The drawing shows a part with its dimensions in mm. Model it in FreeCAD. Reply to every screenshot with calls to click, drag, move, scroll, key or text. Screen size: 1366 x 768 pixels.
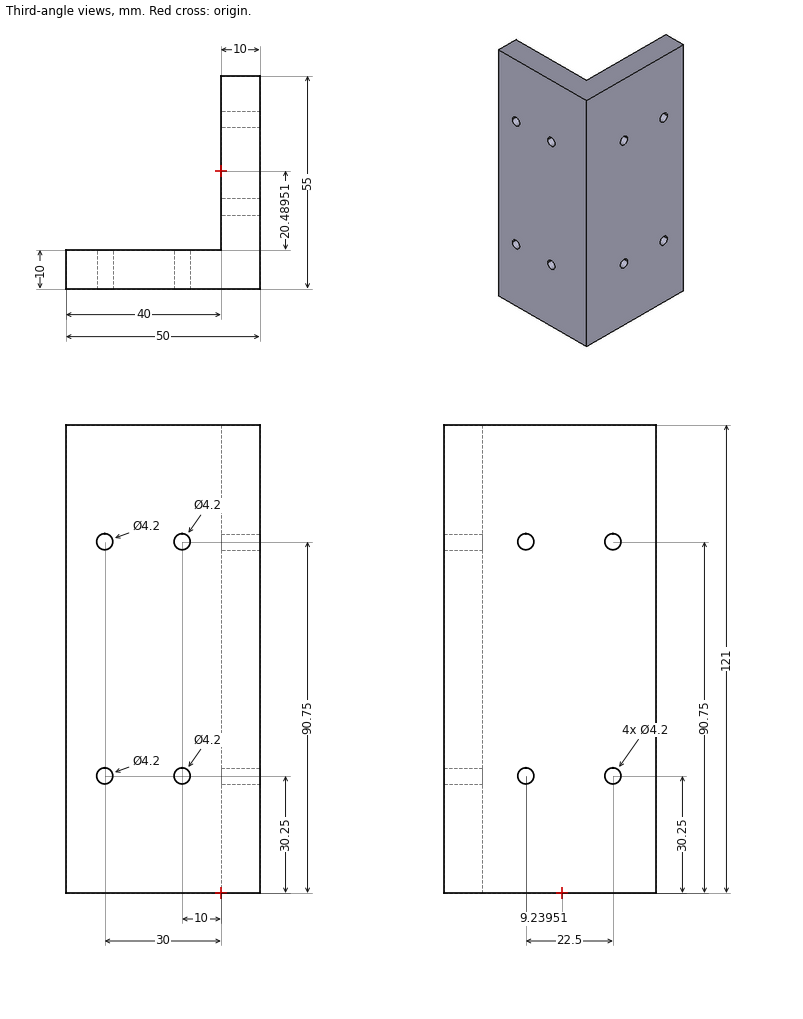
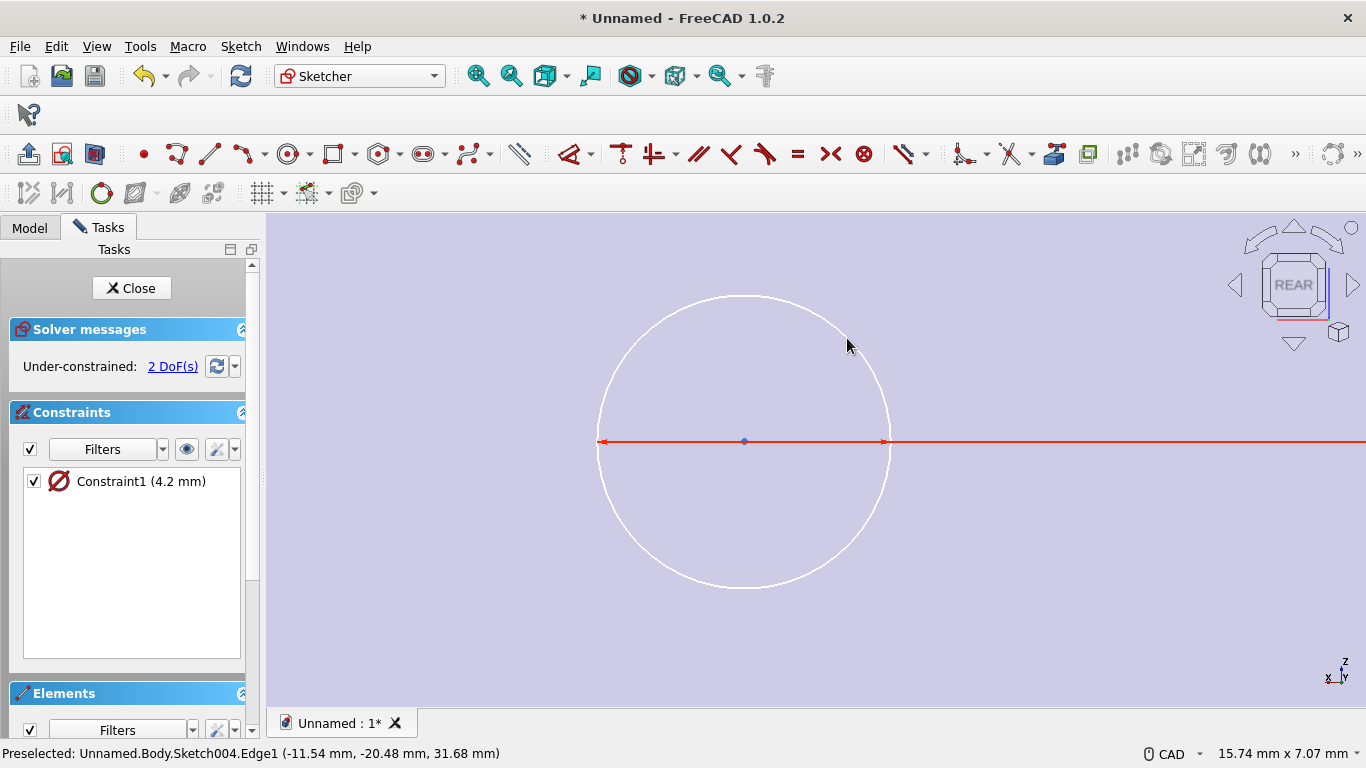
key(d)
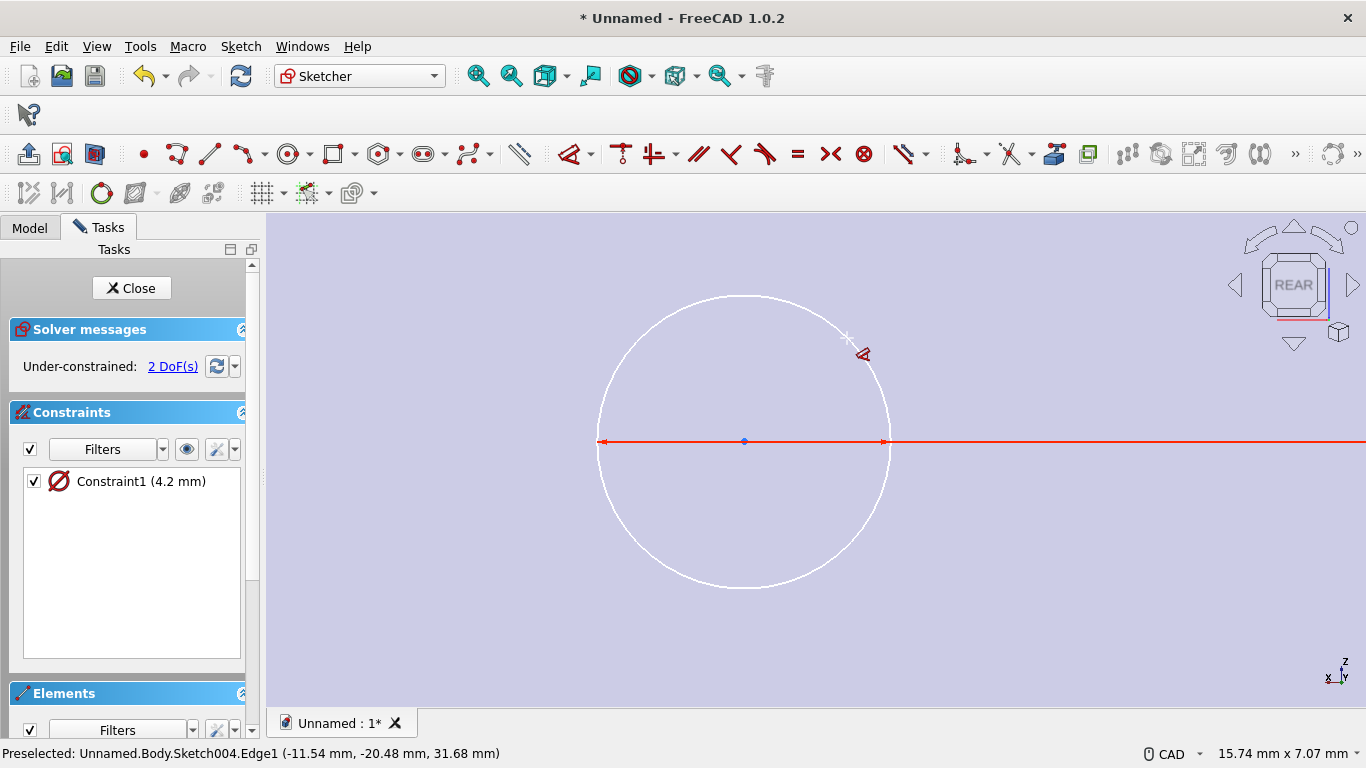
click(744, 442)
click(519, 408)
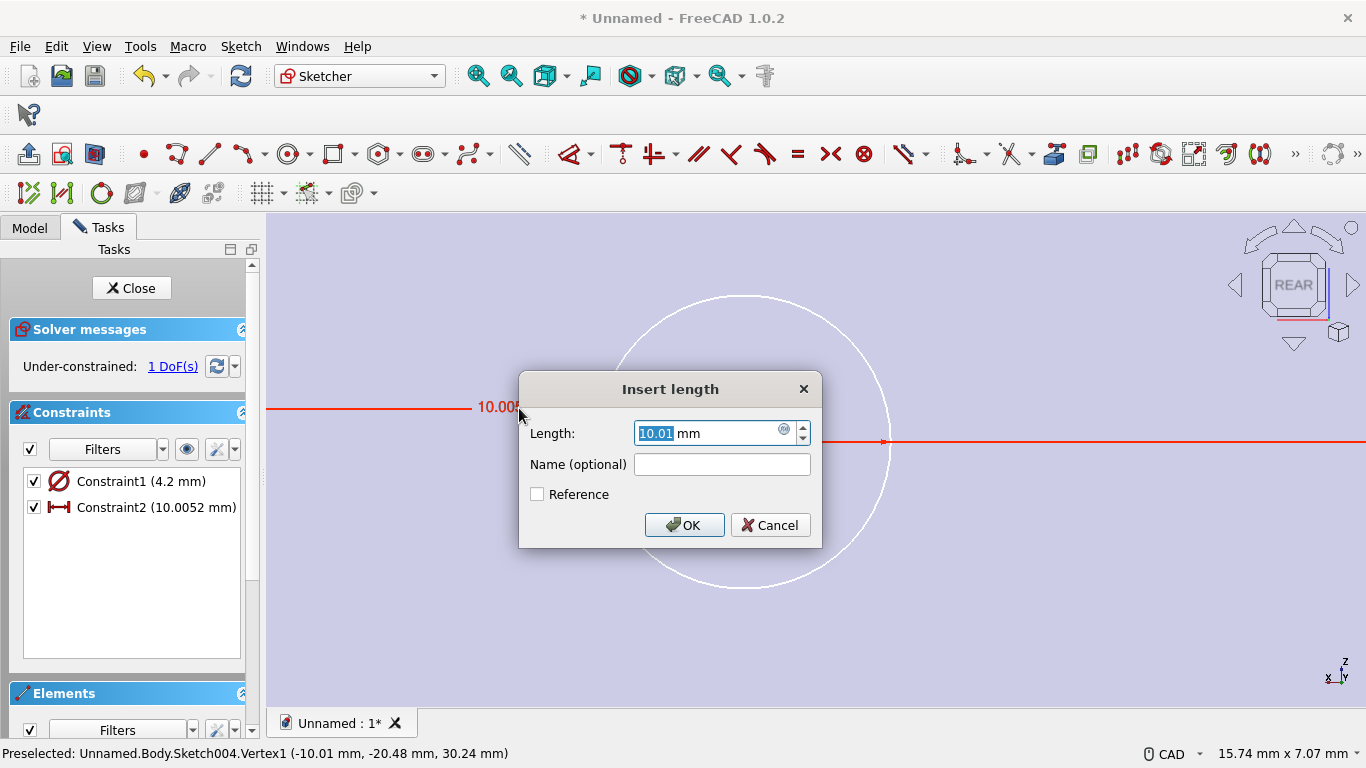
text(10)
key(Return)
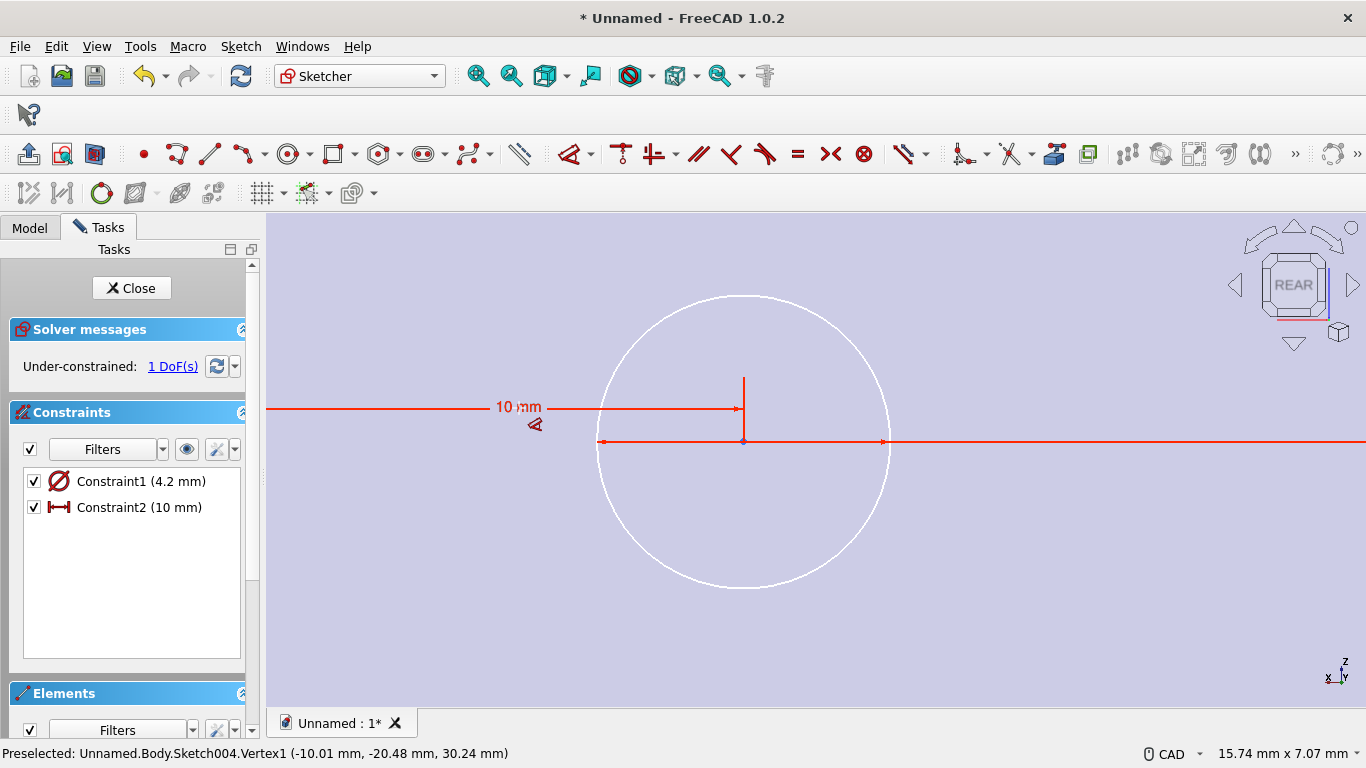
click(744, 442)
click(778, 561)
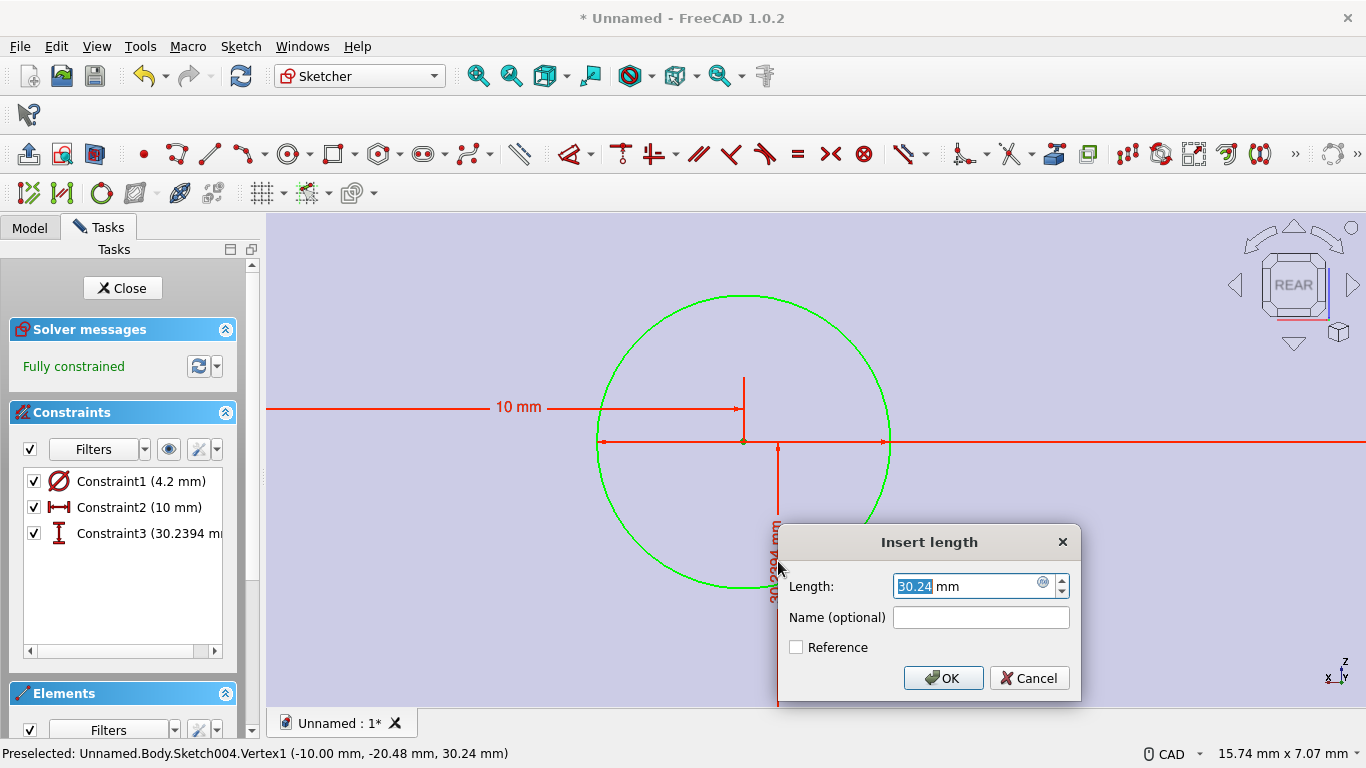
text(30.25)
key(Return)
key(Escape)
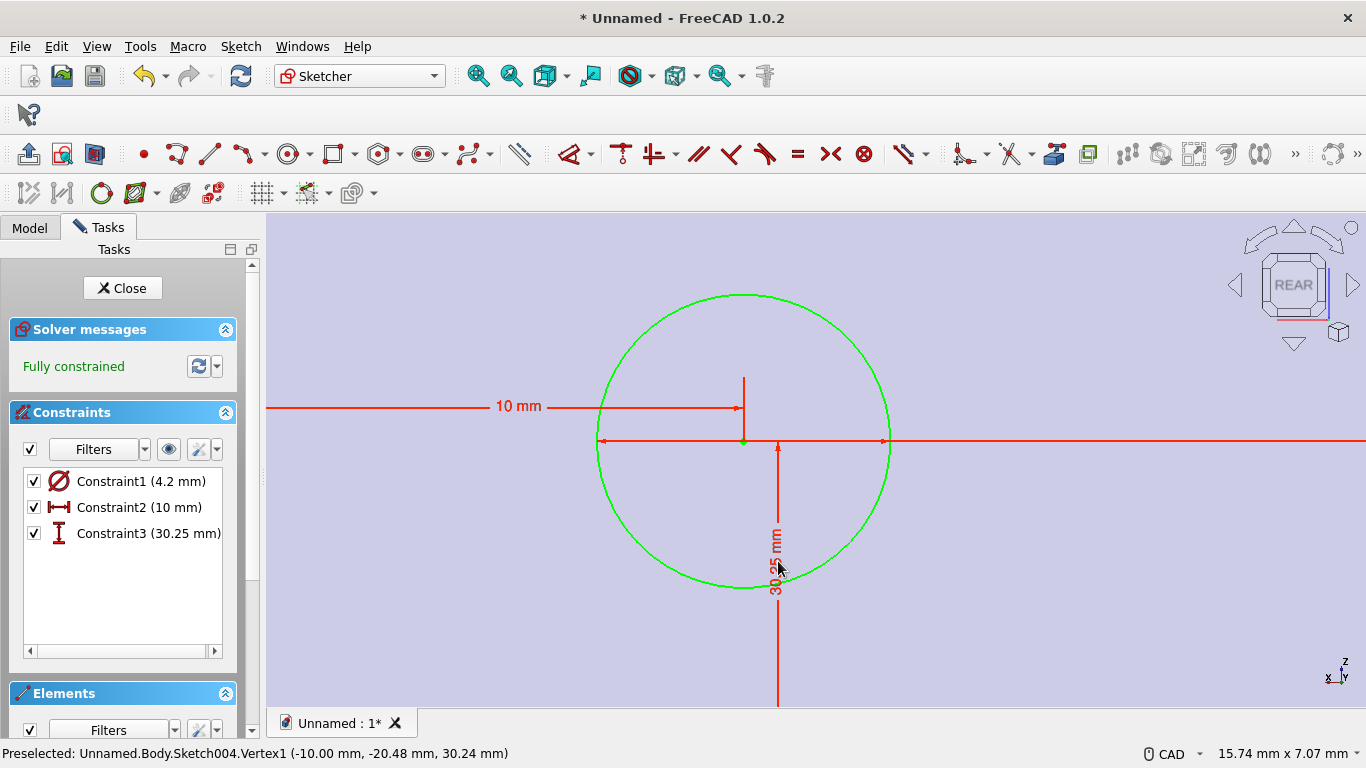
click(123, 288)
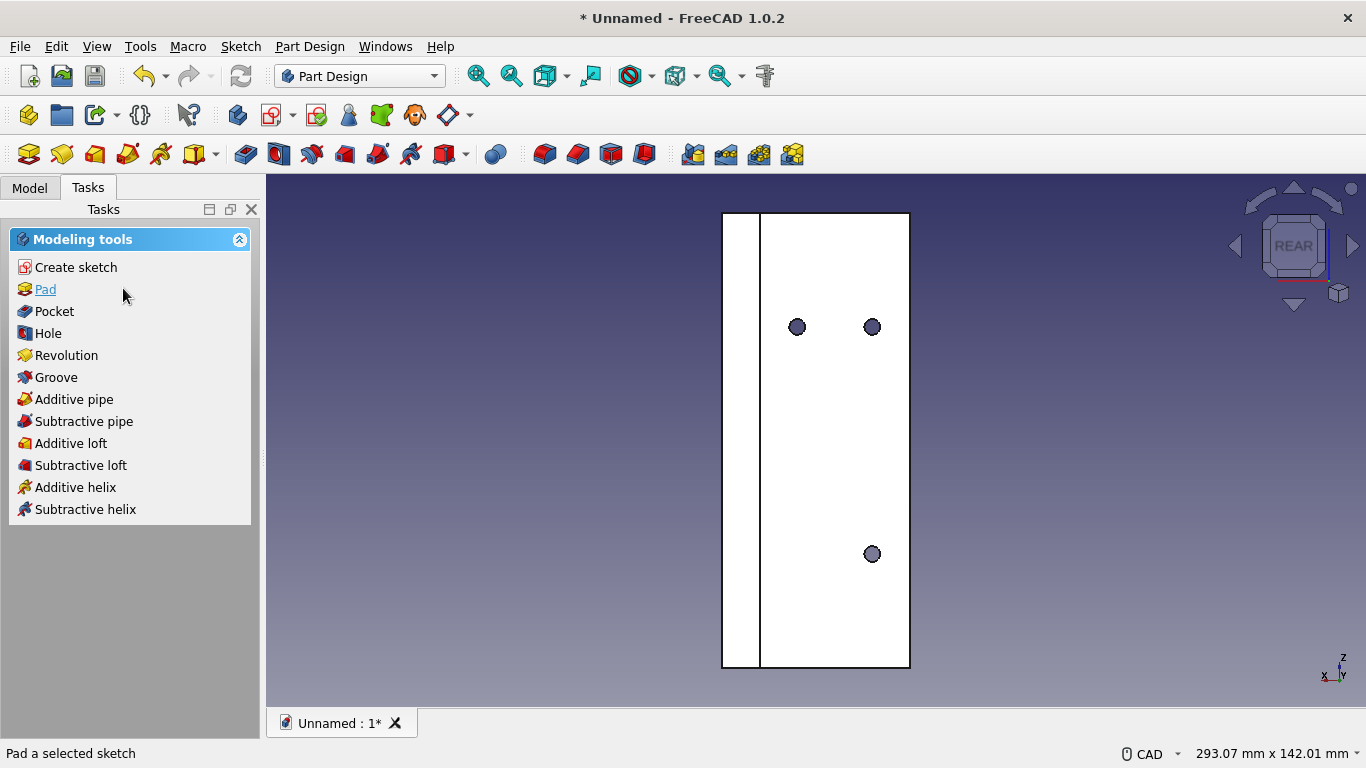
click(246, 154)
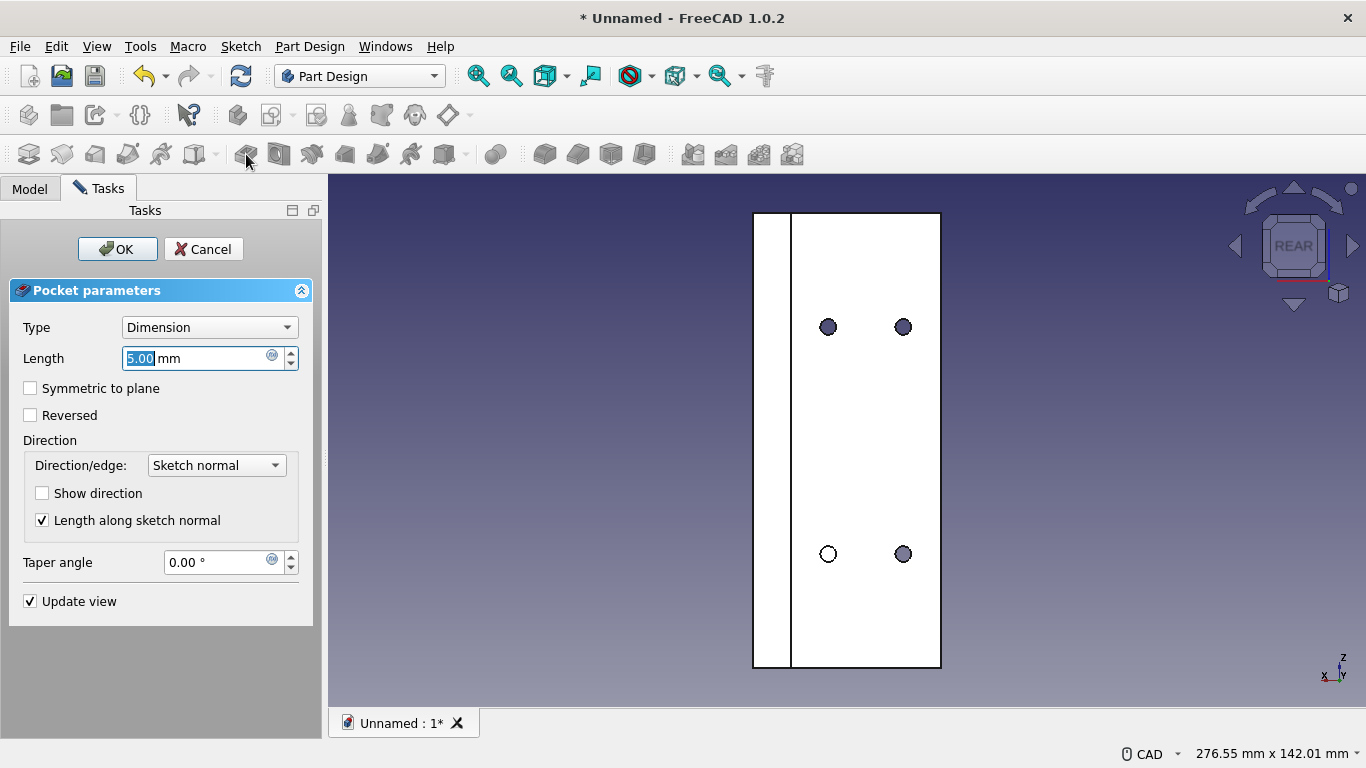
click(210, 328)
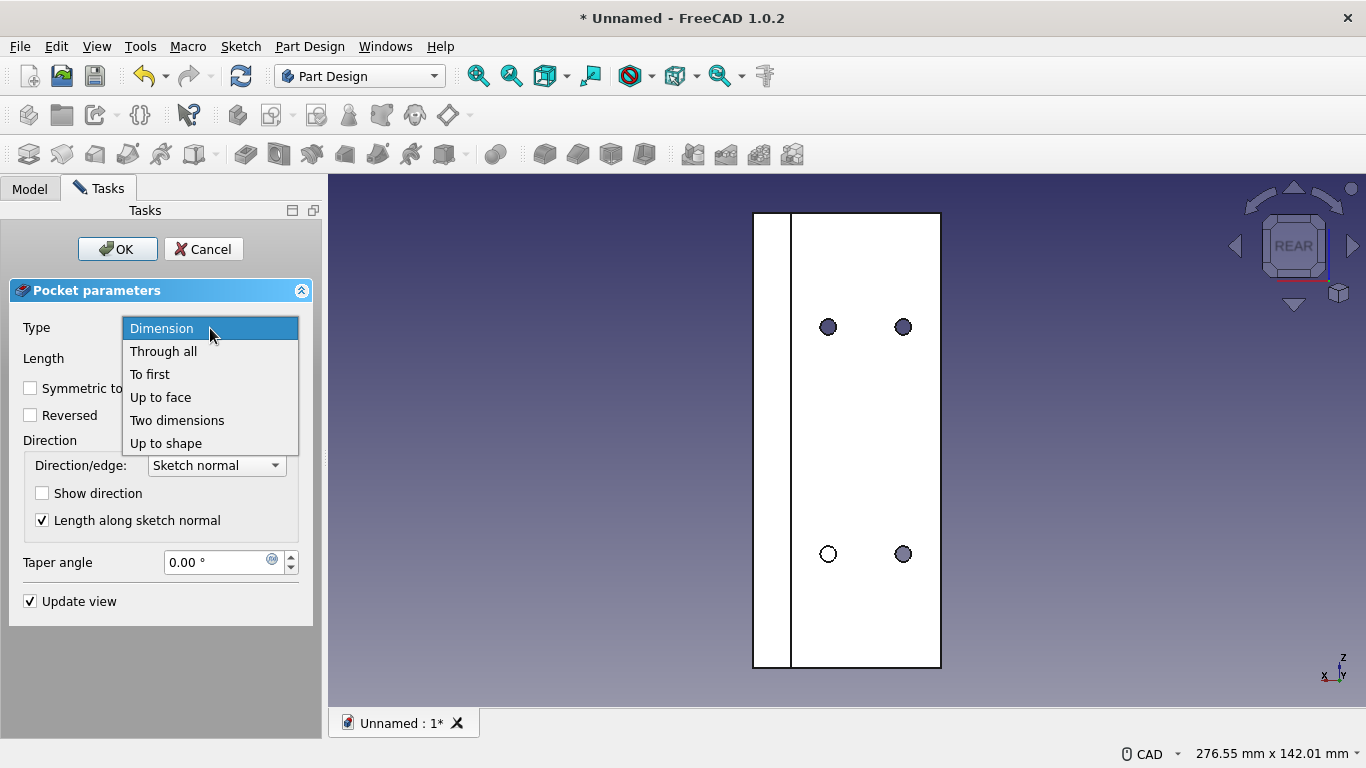
click(208, 374)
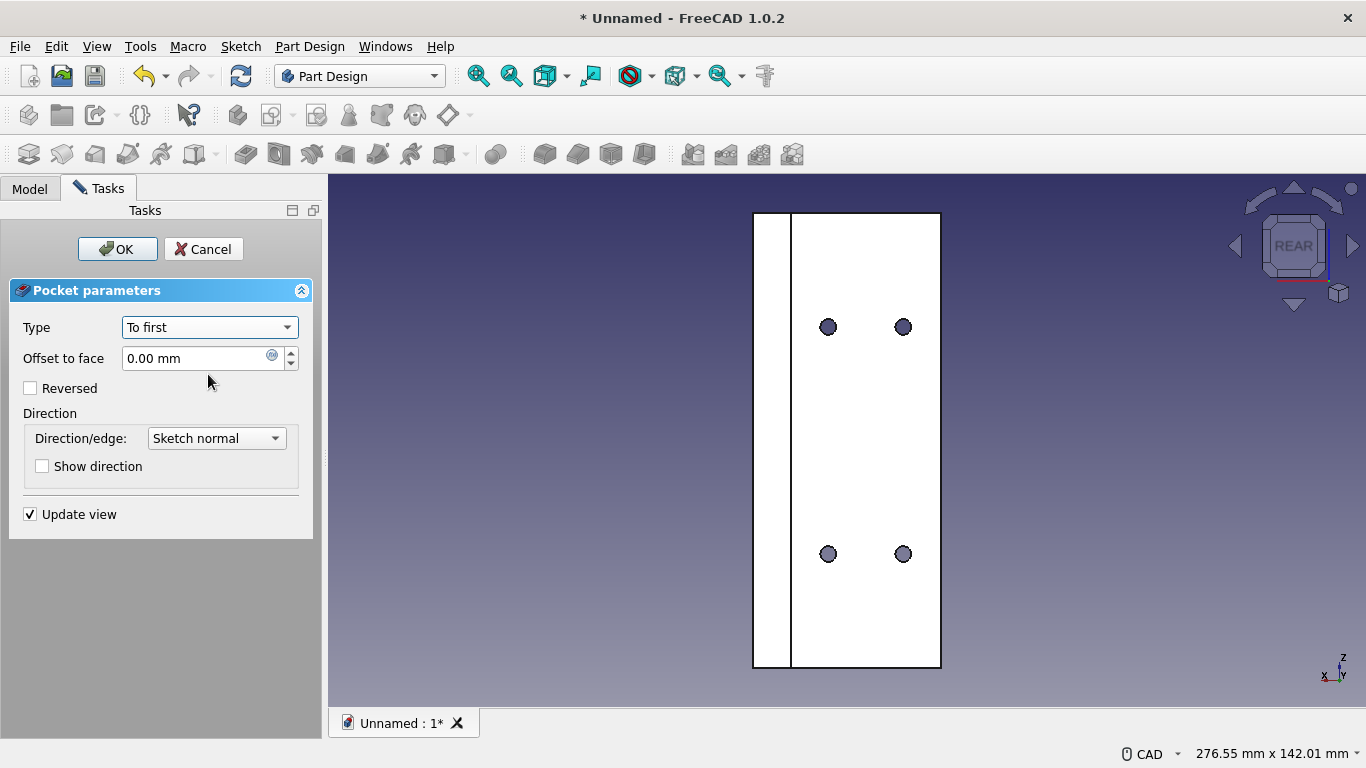
click(118, 249)